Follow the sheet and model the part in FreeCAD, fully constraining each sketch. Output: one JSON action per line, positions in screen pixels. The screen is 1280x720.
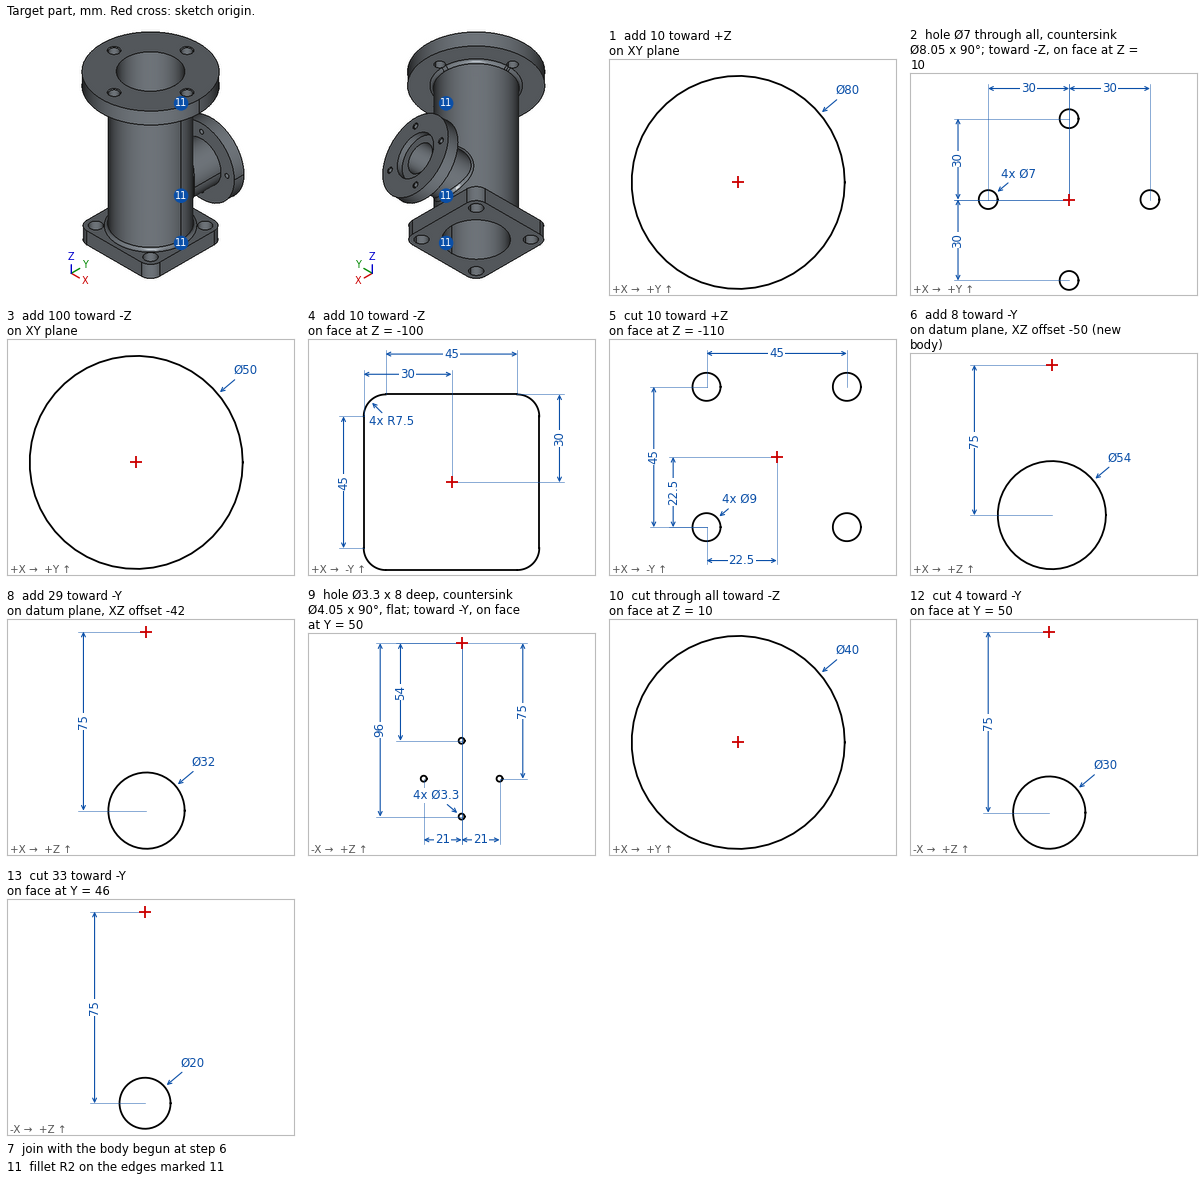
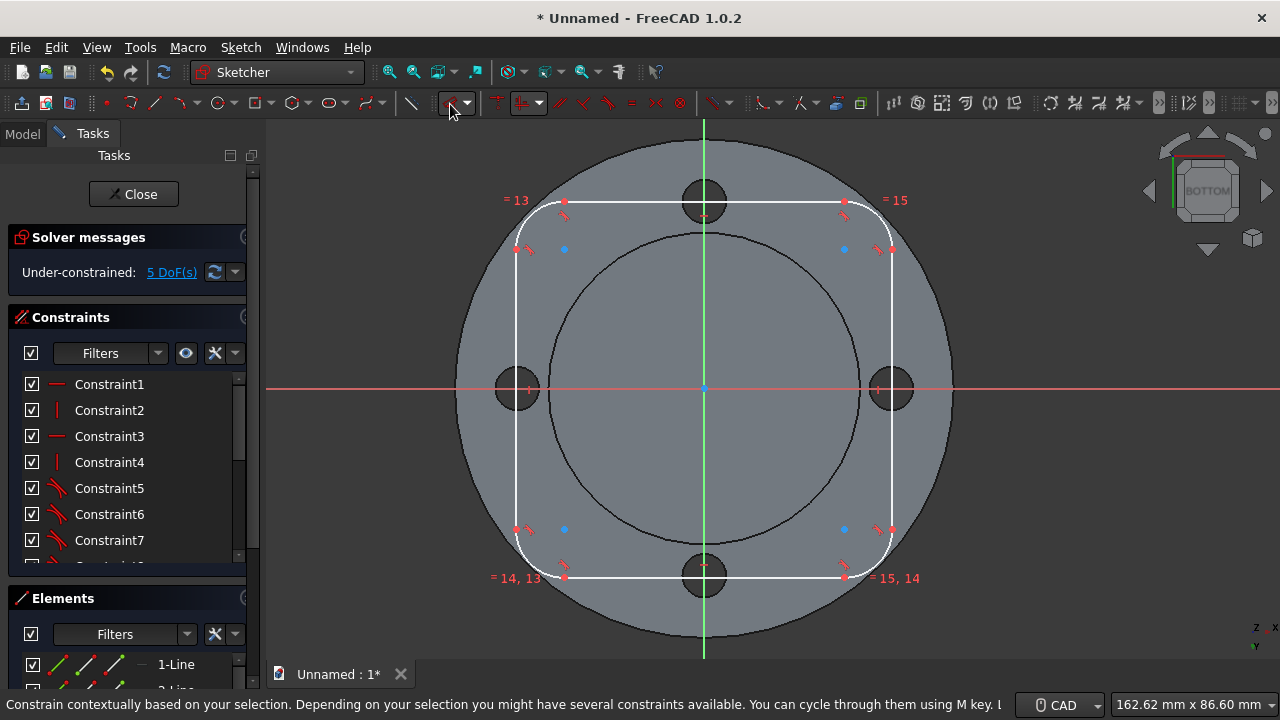
{"action": "left_click", "coordinate": [542, 207]}
{"action": "left_click", "coordinate": [527, 179]}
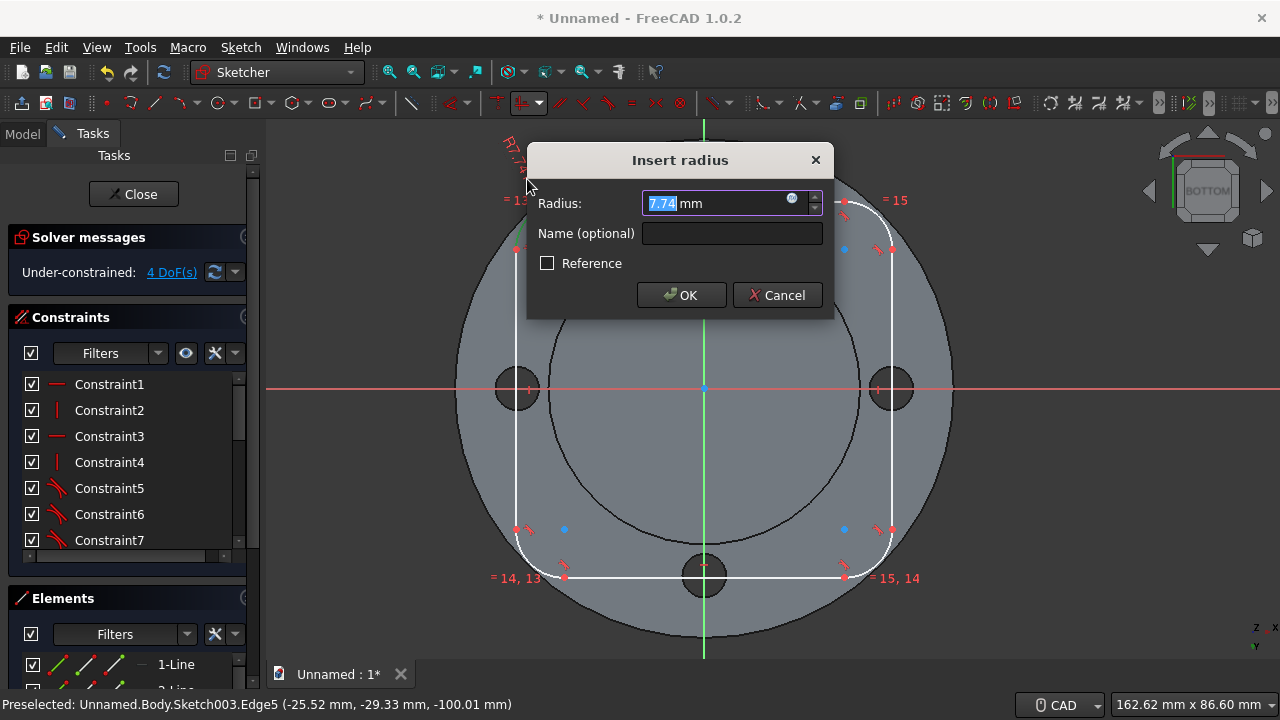
{"action": "type", "text": "7.5"}
{"action": "key", "text": "Return"}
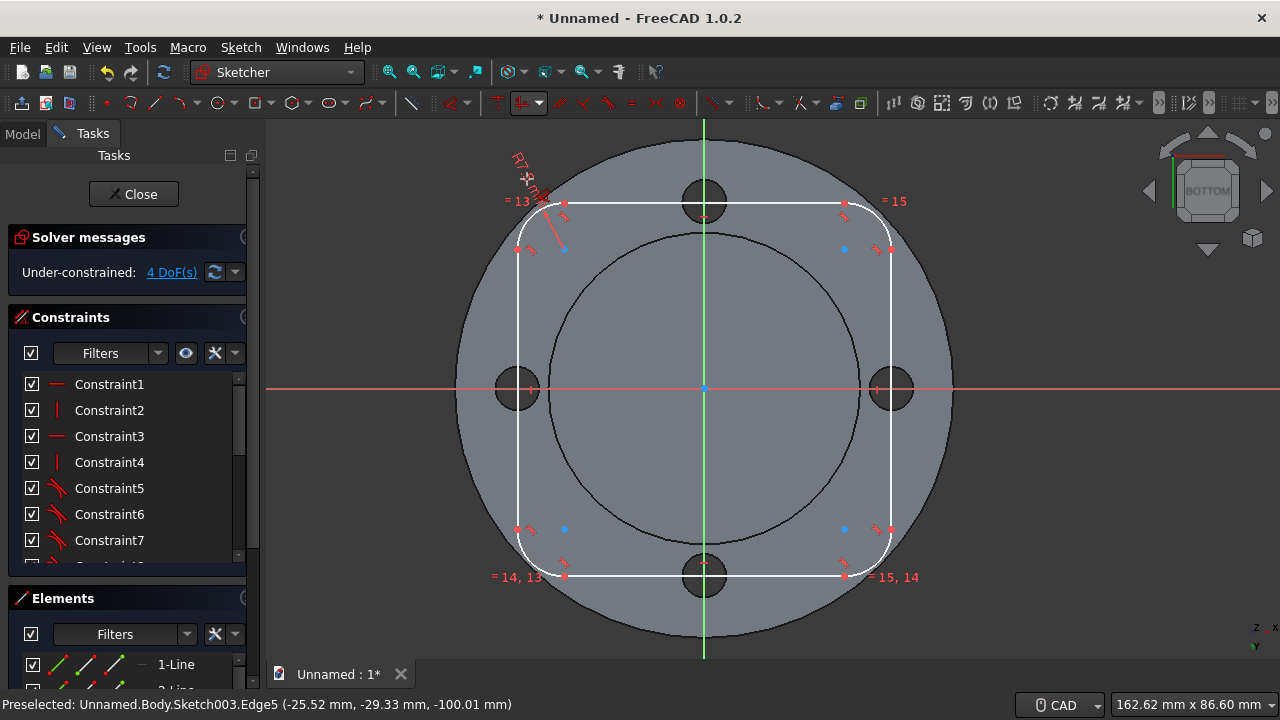
{"action": "left_click", "coordinate": [761, 203]}
{"action": "left_click", "coordinate": [640, 169]}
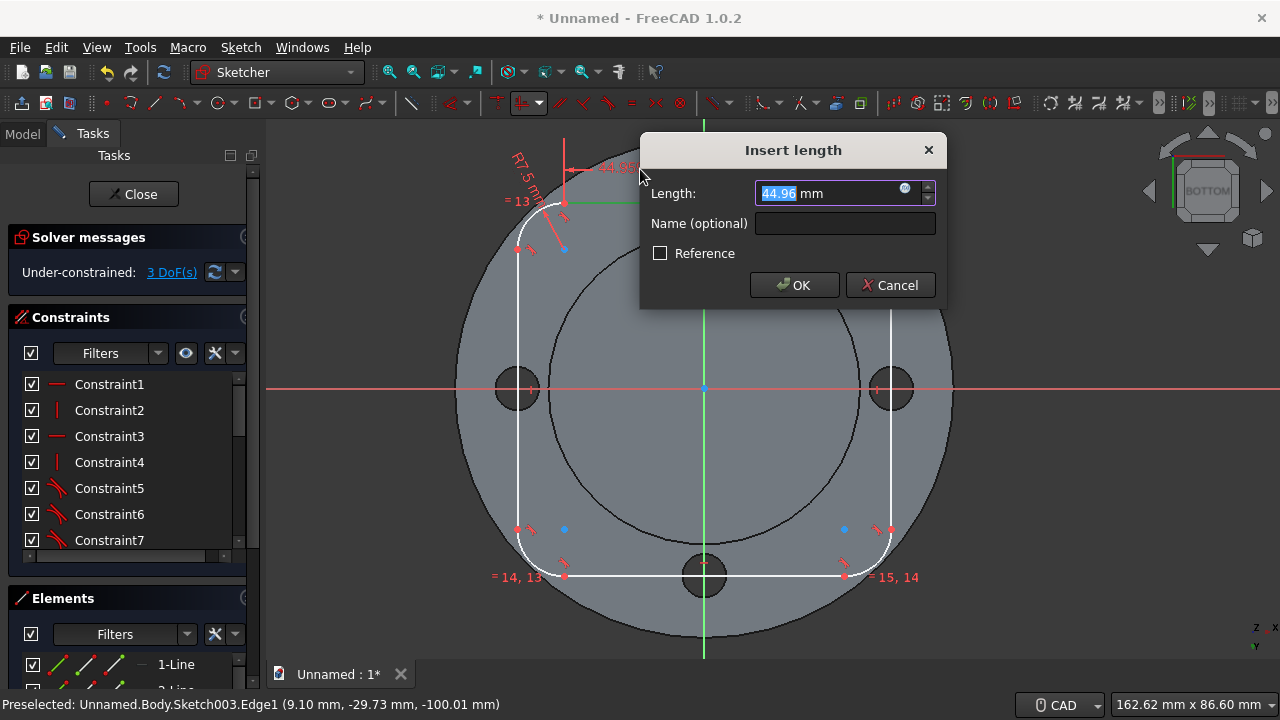
{"action": "type", "text": "45"}
{"action": "key", "text": "Return"}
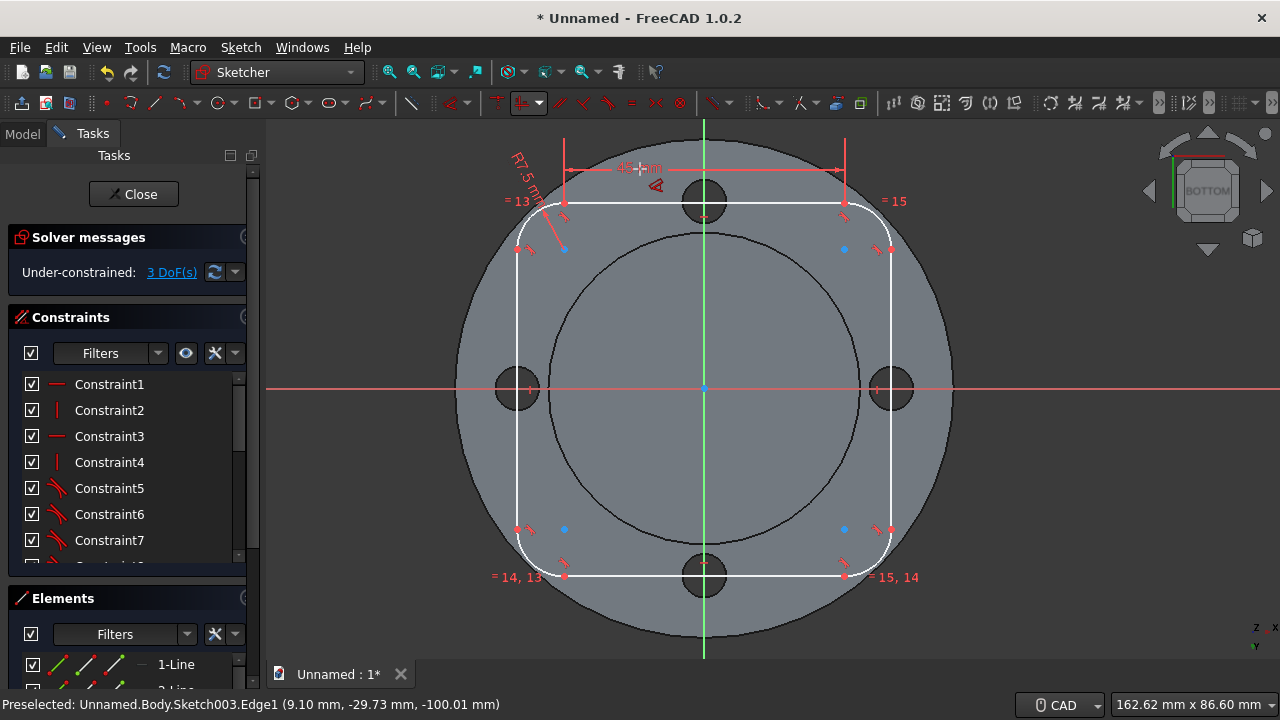
{"action": "left_click", "coordinate": [517, 334]}
{"action": "left_click", "coordinate": [483, 325]}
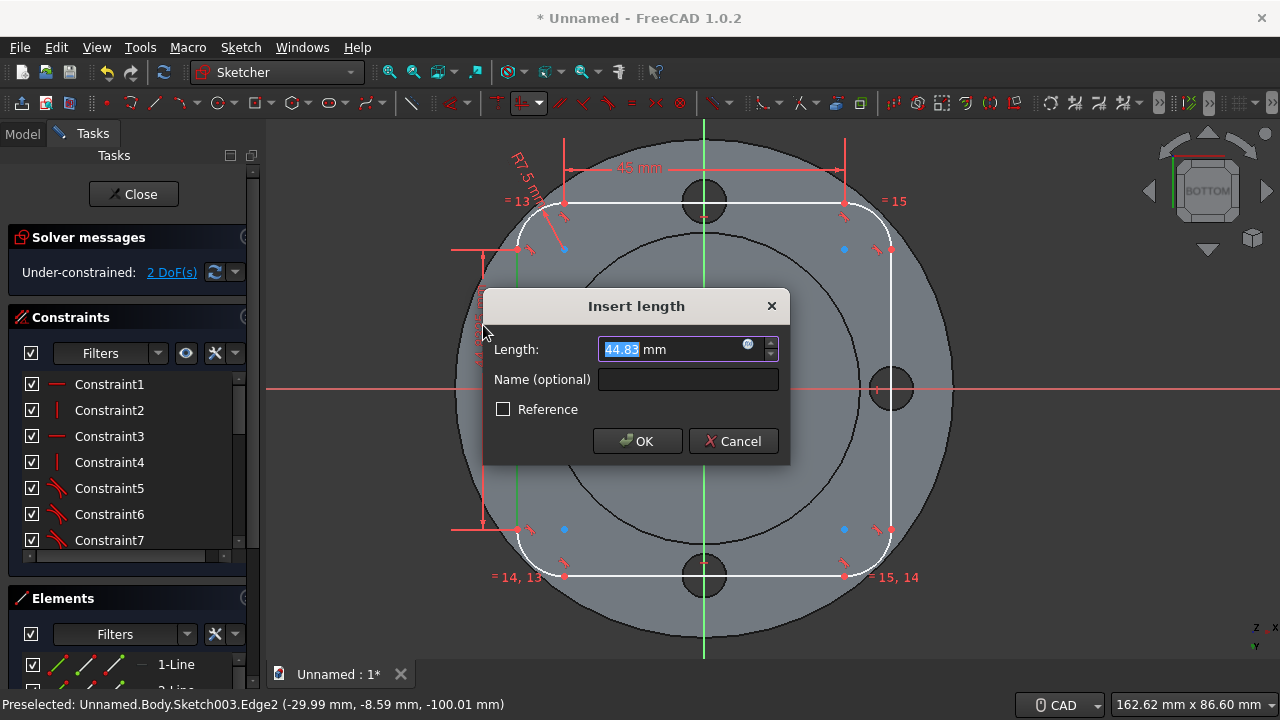
{"action": "type", "text": "45"}
{"action": "key", "text": "Return"}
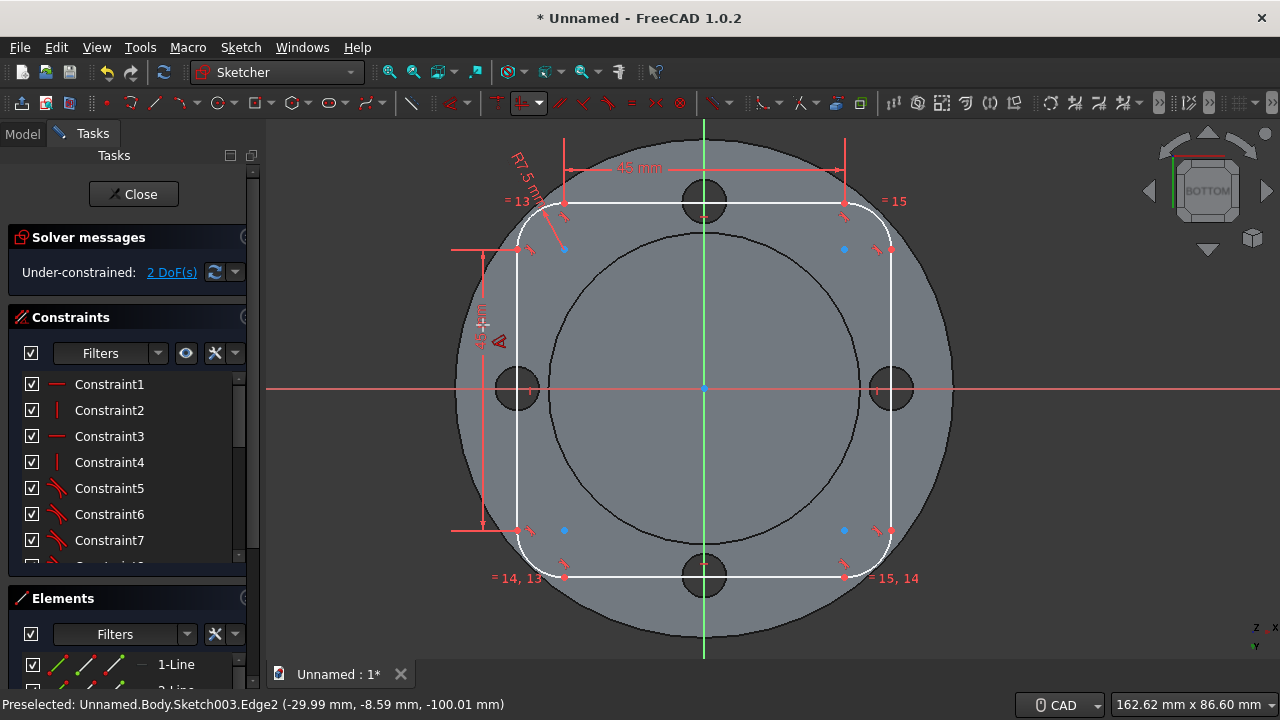
{"action": "left_click", "coordinate": [845, 203]}
{"action": "left_click", "coordinate": [670, 296]}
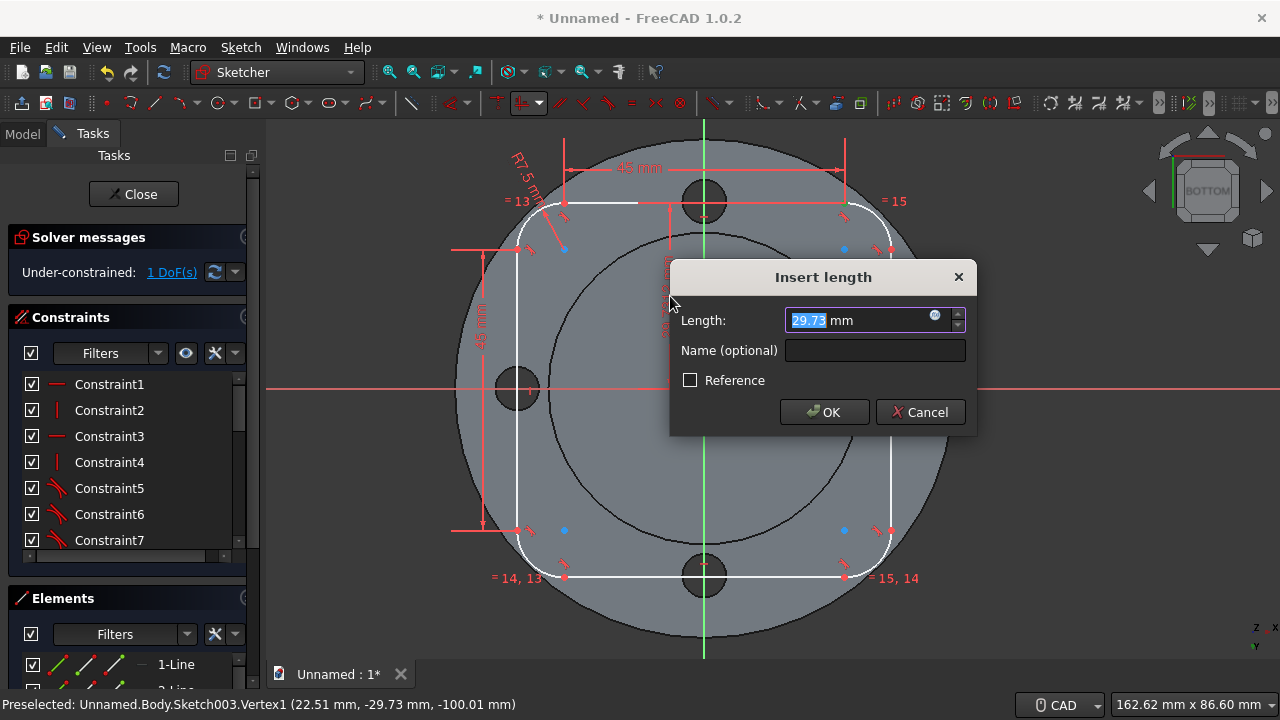
{"action": "type", "text": "30"}
{"action": "key", "text": "Return"}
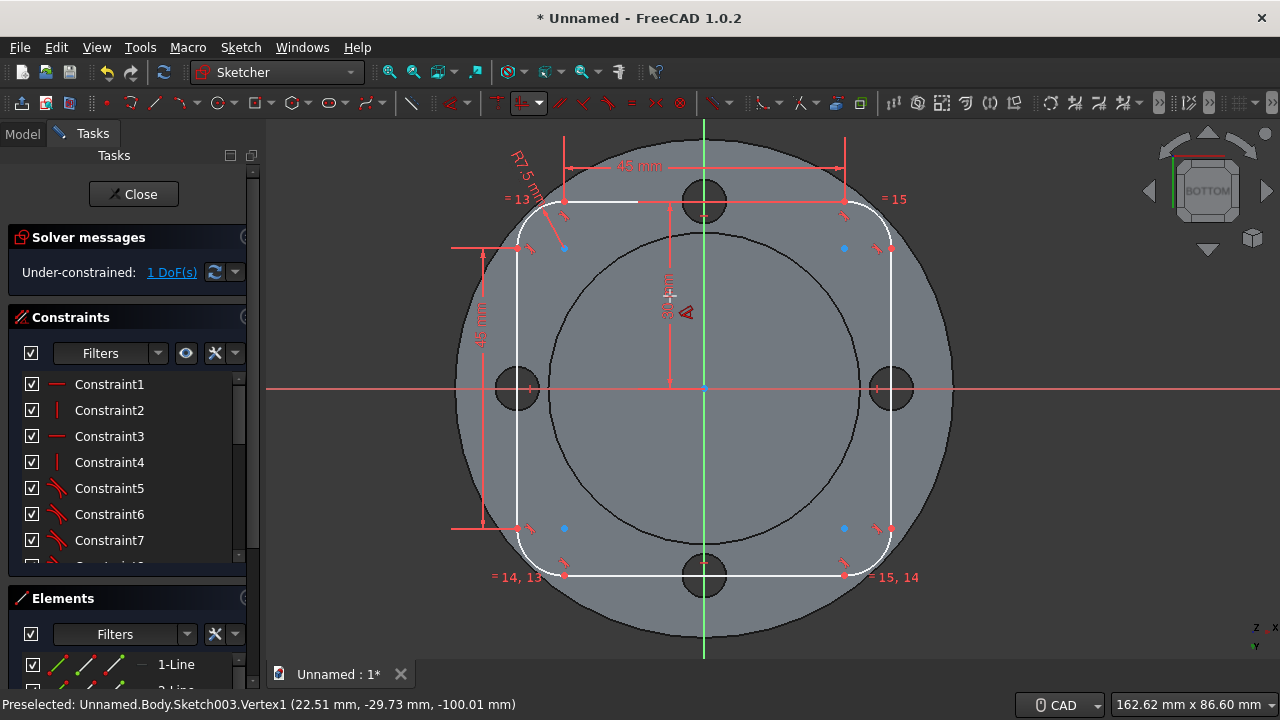
{"action": "left_click", "coordinate": [517, 248]}
{"action": "left_click", "coordinate": [611, 423]}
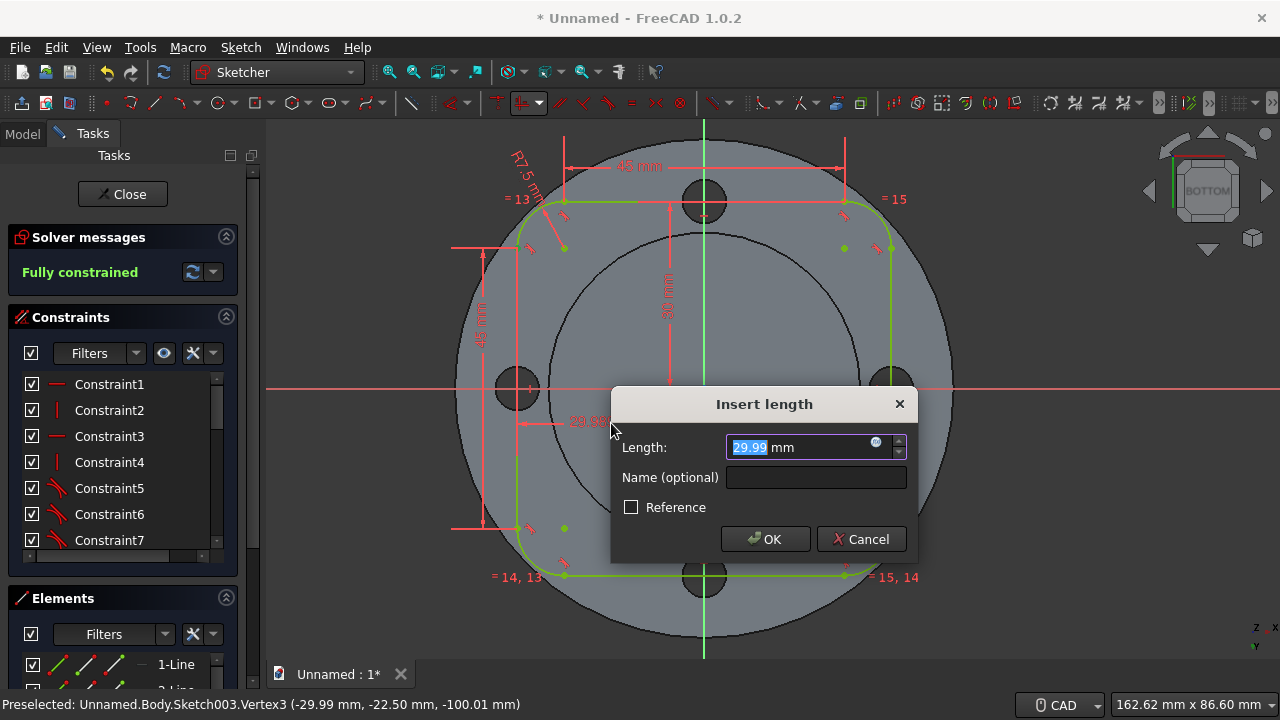
{"action": "type", "text": "30"}
{"action": "key", "text": "Return"}
{"action": "key", "text": "Escape"}